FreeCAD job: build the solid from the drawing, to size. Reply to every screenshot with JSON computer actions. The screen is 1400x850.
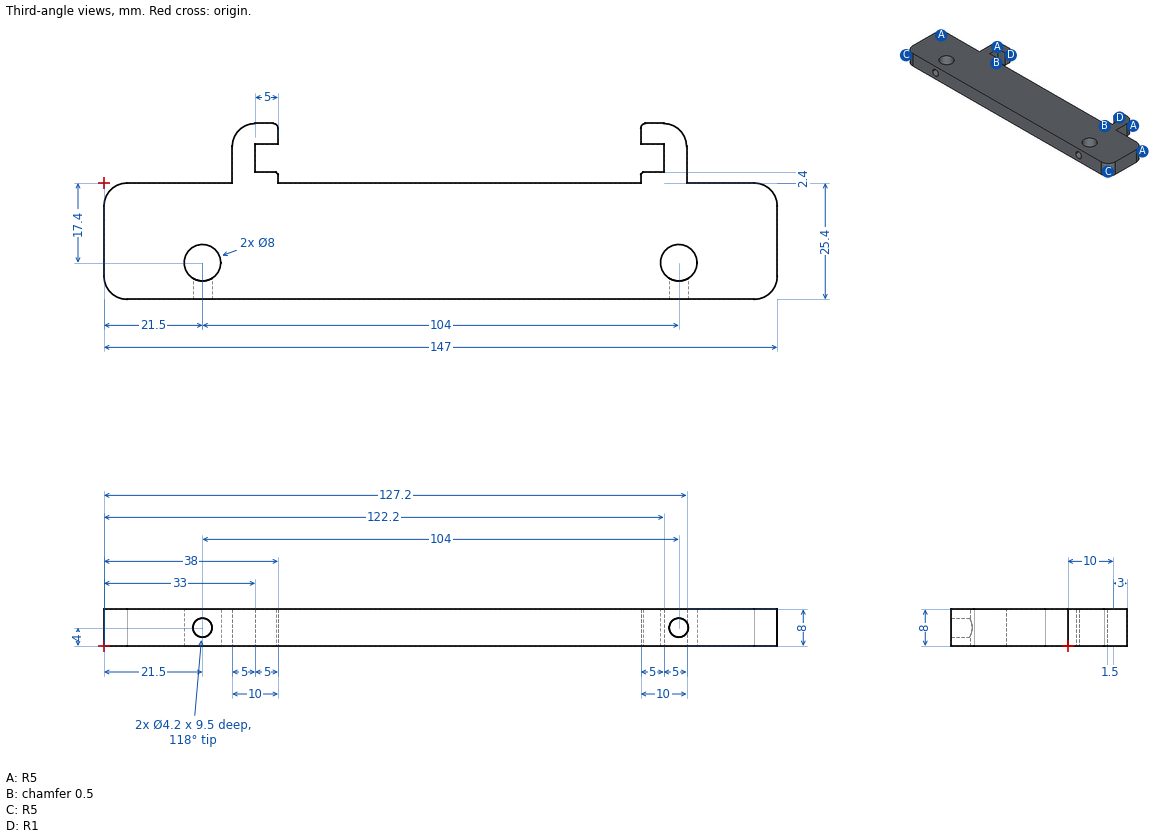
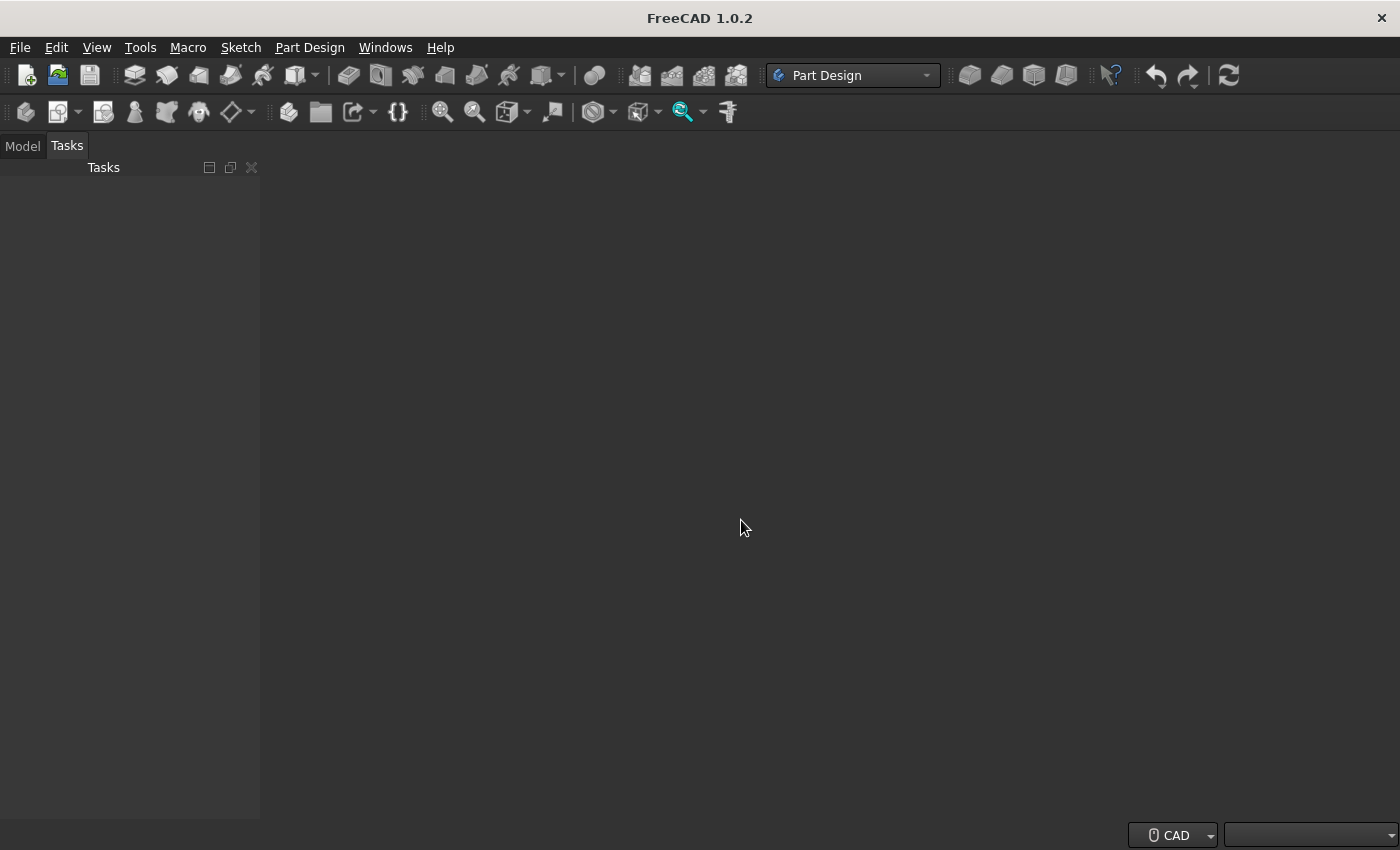
{"action": "left_click", "coordinate": [26, 76]}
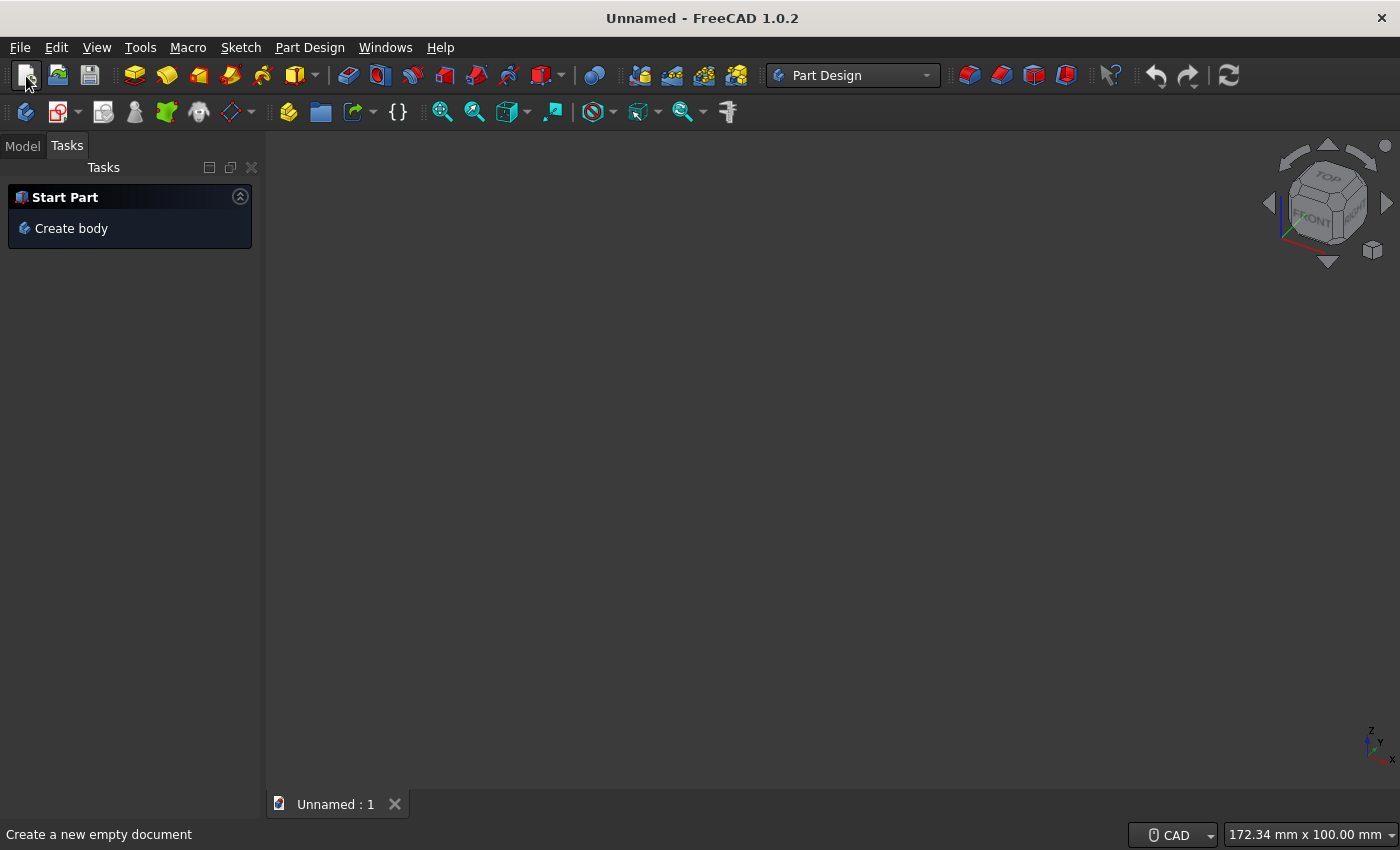
{"action": "left_click", "coordinate": [58, 112]}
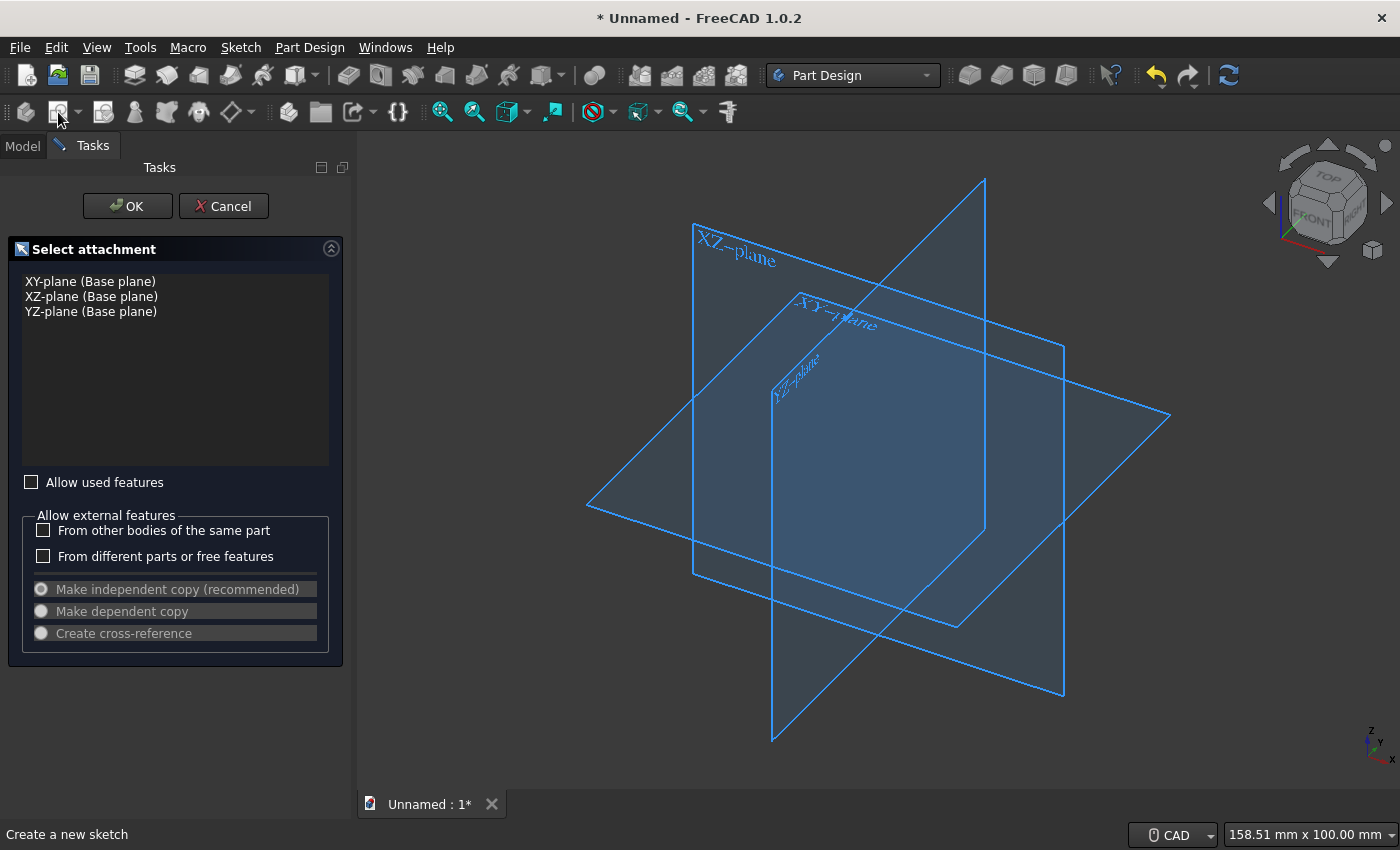
{"action": "left_click", "coordinate": [82, 282]}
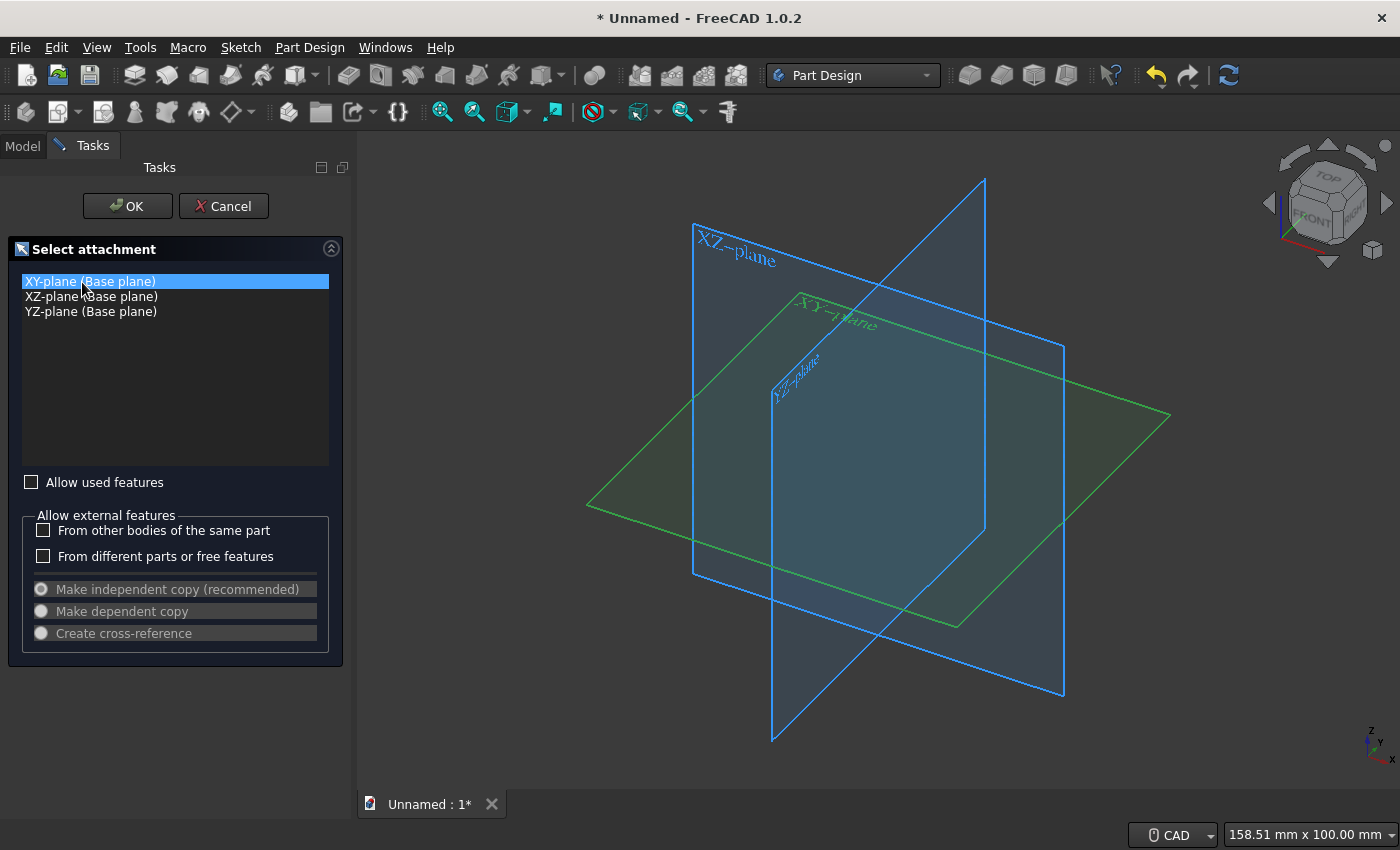
{"action": "left_click", "coordinate": [128, 206]}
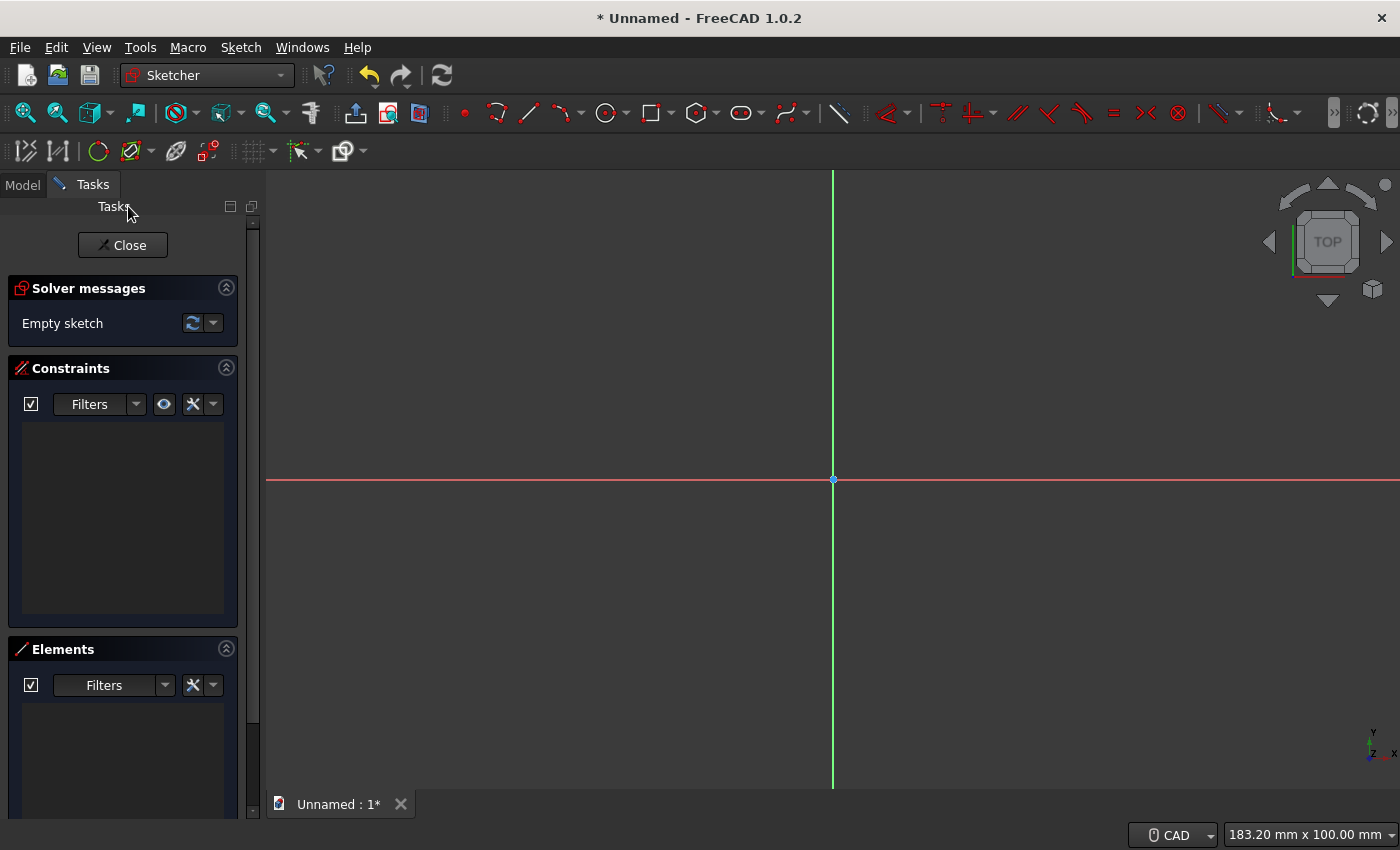
{"action": "scroll", "coordinate": [294, 384], "scroll_direction": "down", "scroll_amount": 3}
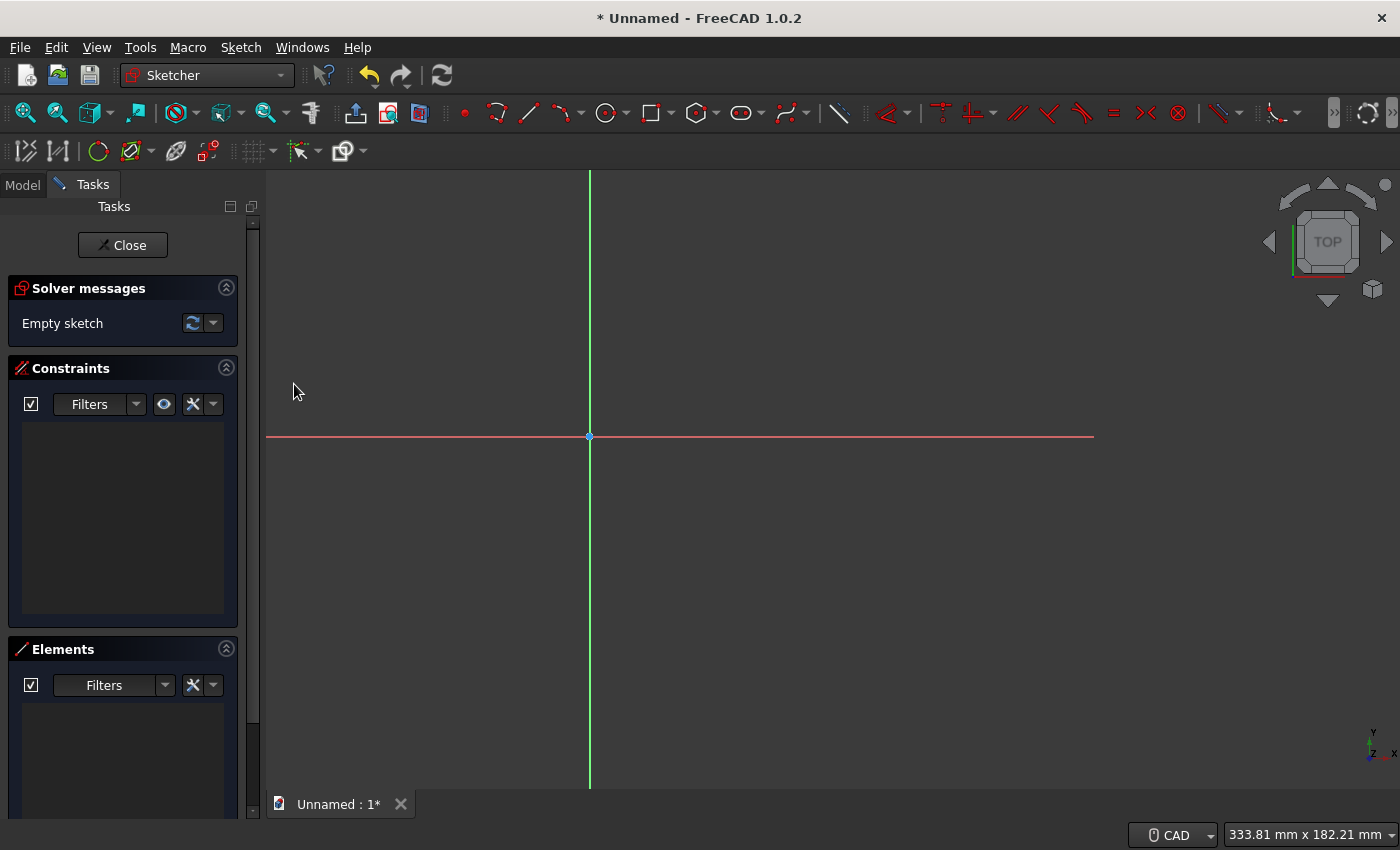
{"action": "left_click", "coordinate": [652, 114]}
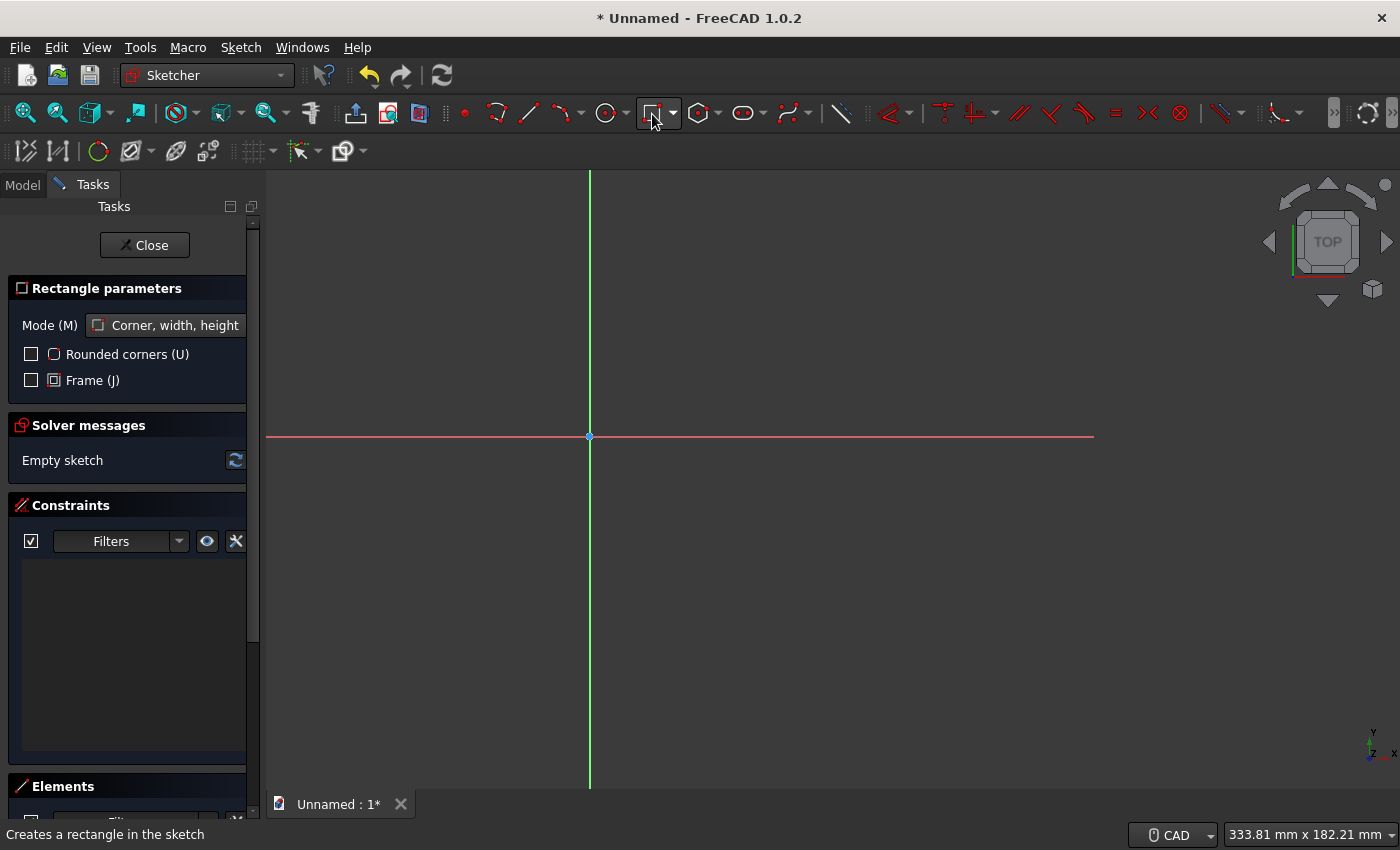
{"action": "left_click", "coordinate": [590, 437]}
{"action": "mouse_move", "coordinate": [1089, 523]}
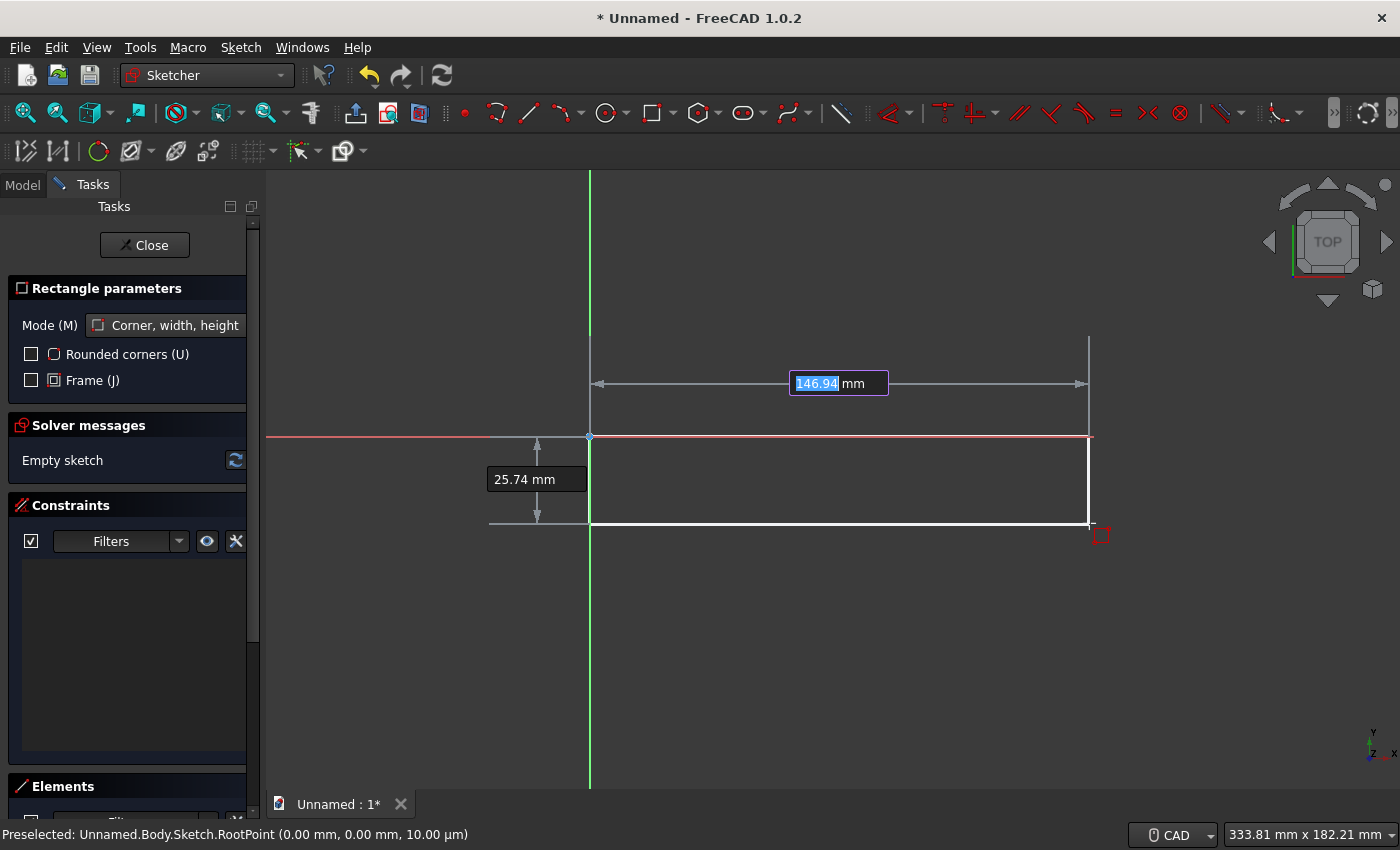
{"action": "type", "text": "147"}
{"action": "key", "text": "Tab"}
{"action": "type", "text": "25.4"}
{"action": "key", "text": "Return"}
{"action": "key", "text": "Escape"}